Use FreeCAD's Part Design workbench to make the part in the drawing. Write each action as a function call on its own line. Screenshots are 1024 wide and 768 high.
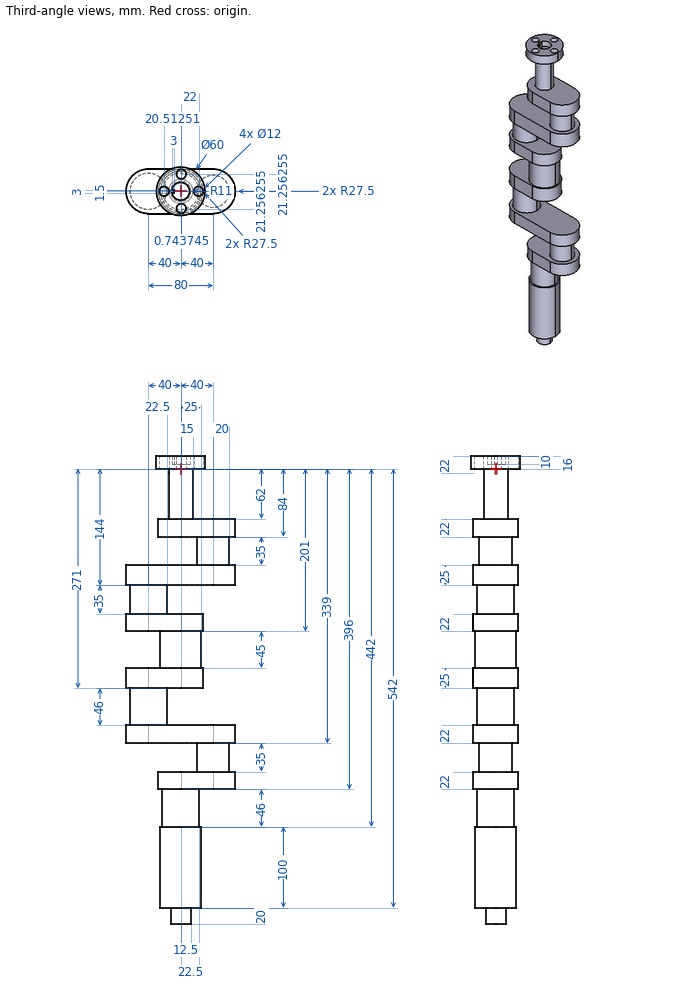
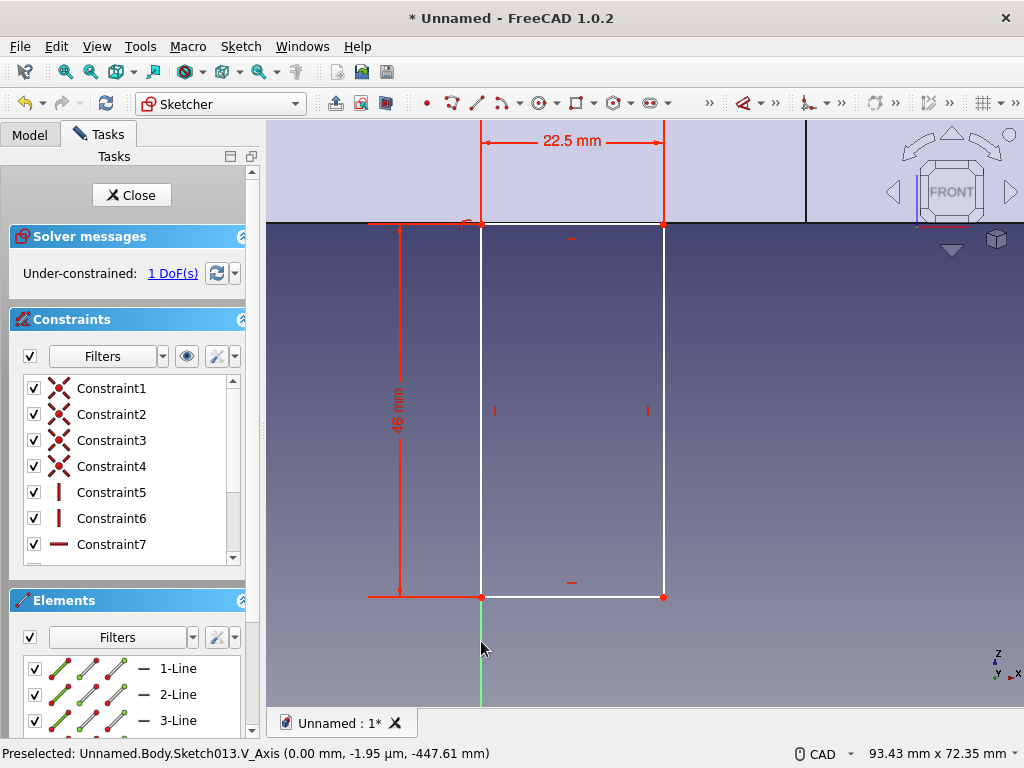
click(742, 104)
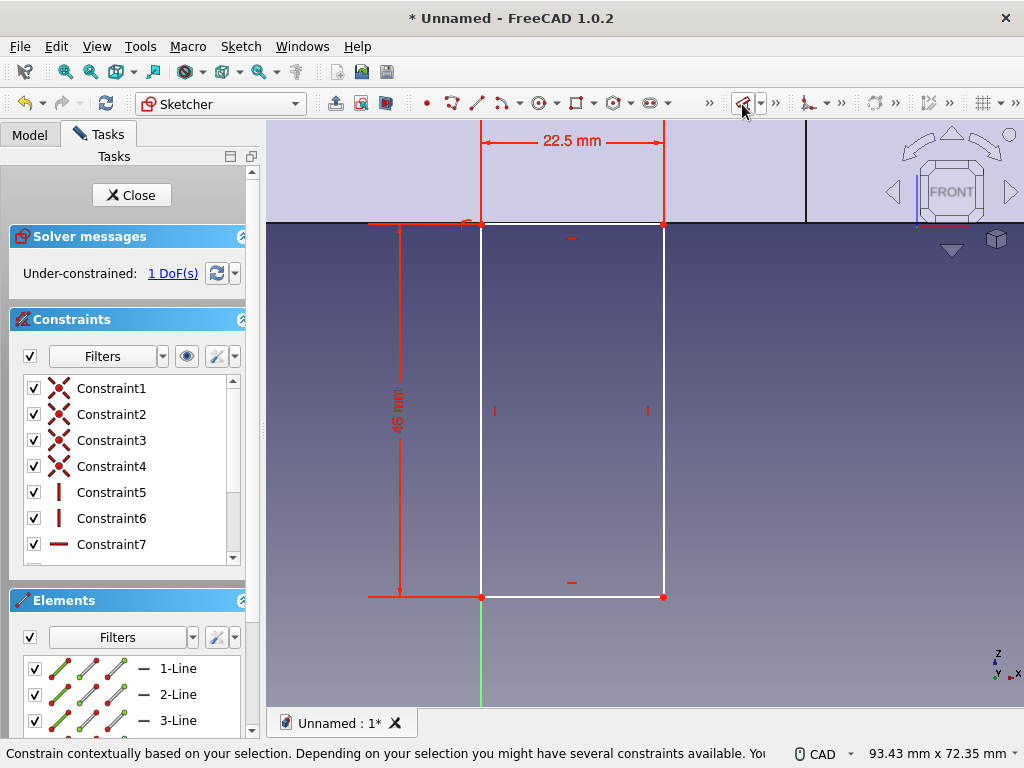
click(481, 224)
click(447, 186)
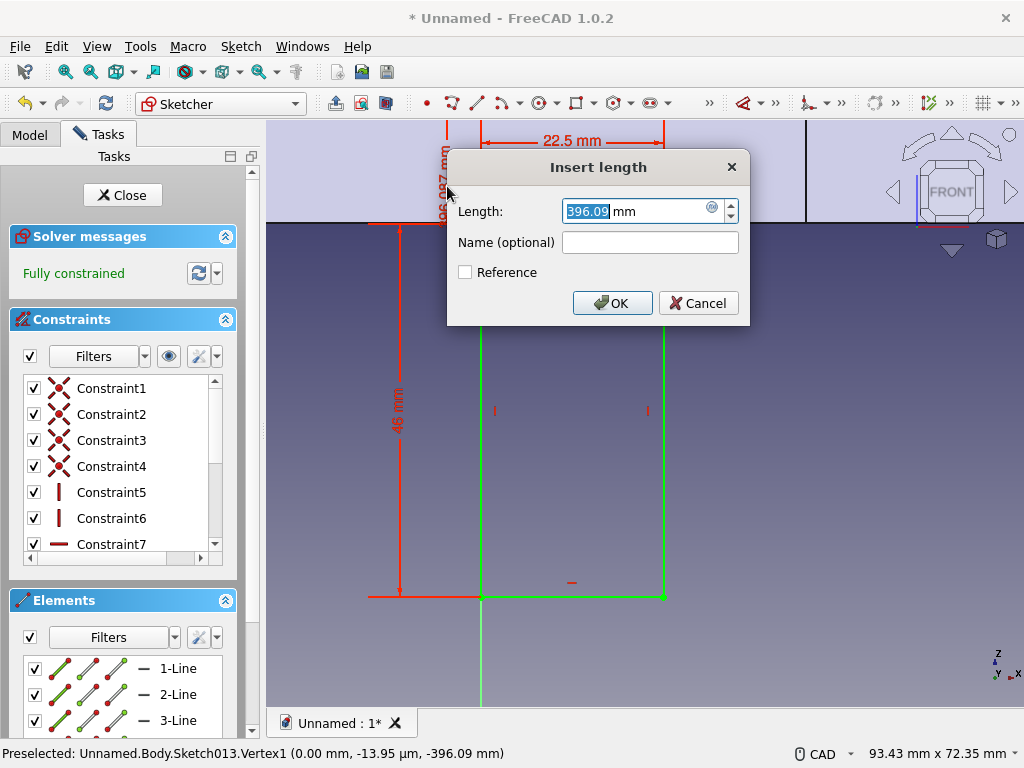
text(396)
key(Return)
key(Escape)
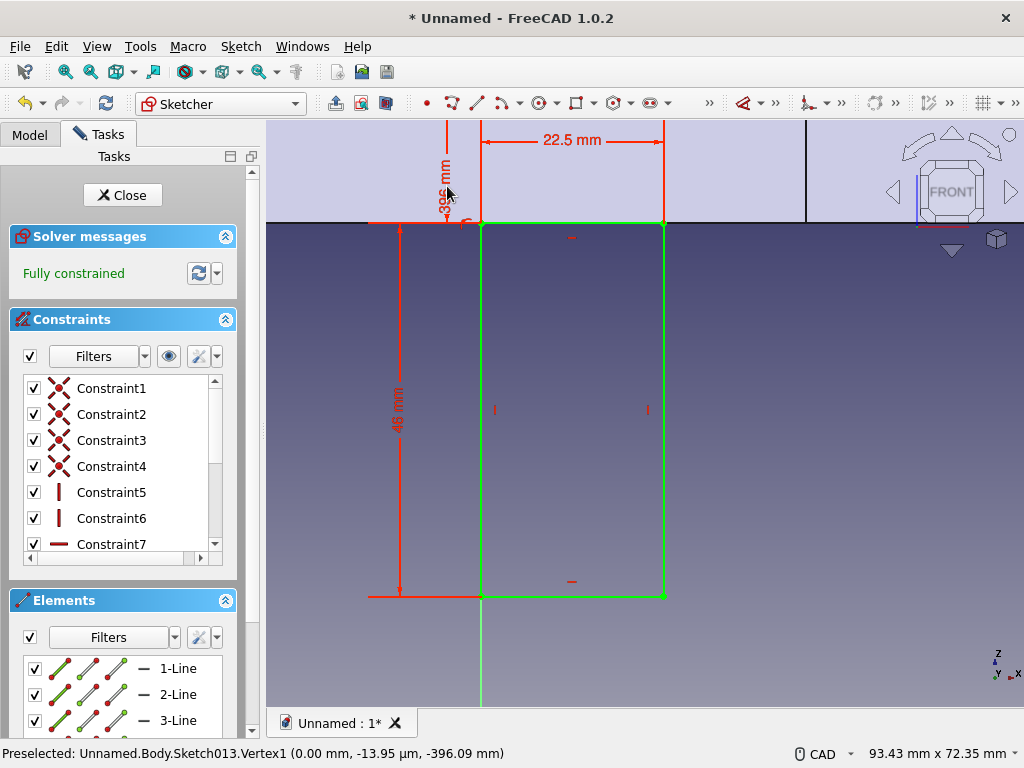
click(123, 195)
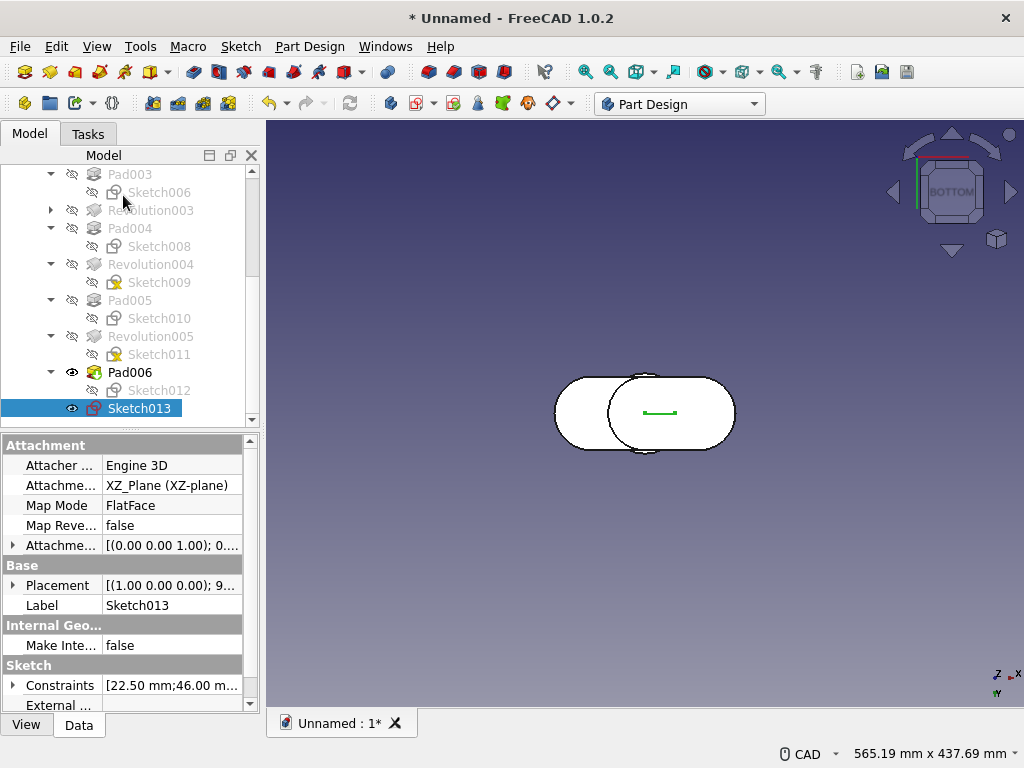
click(50, 72)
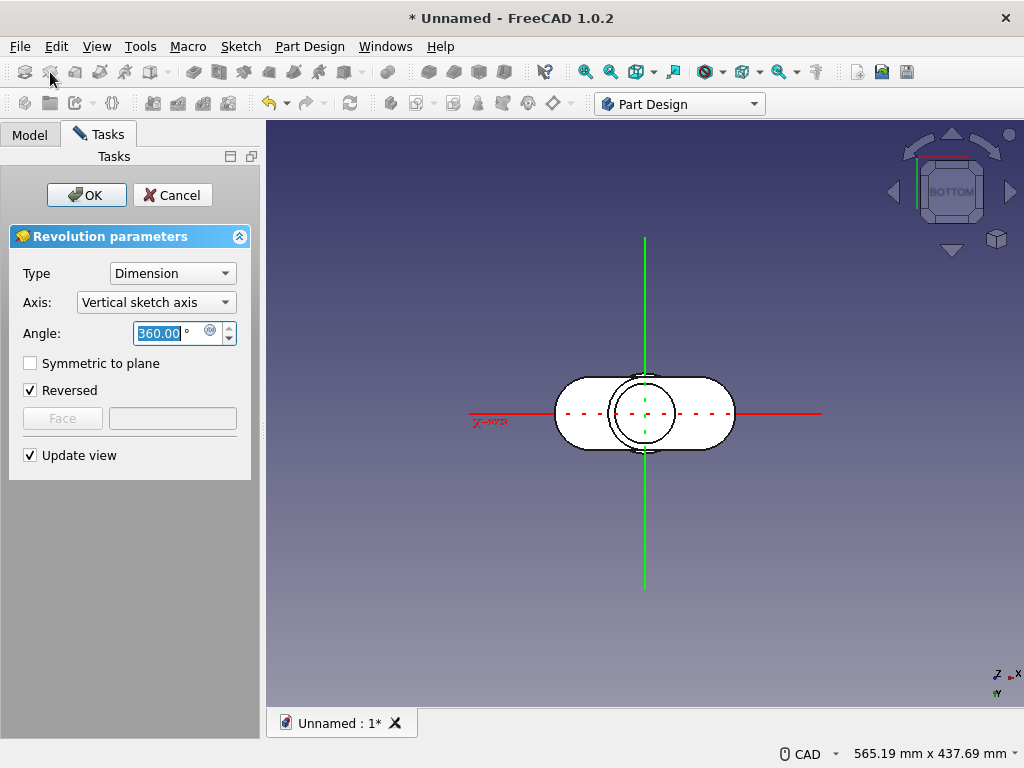
click(87, 195)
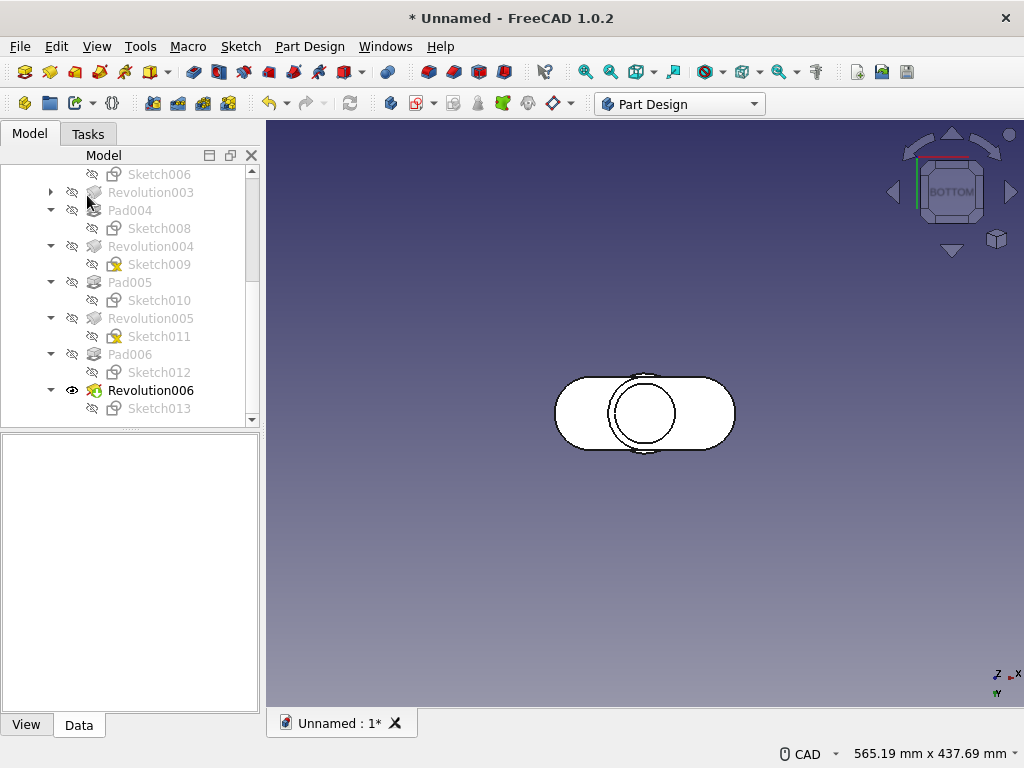
click(586, 72)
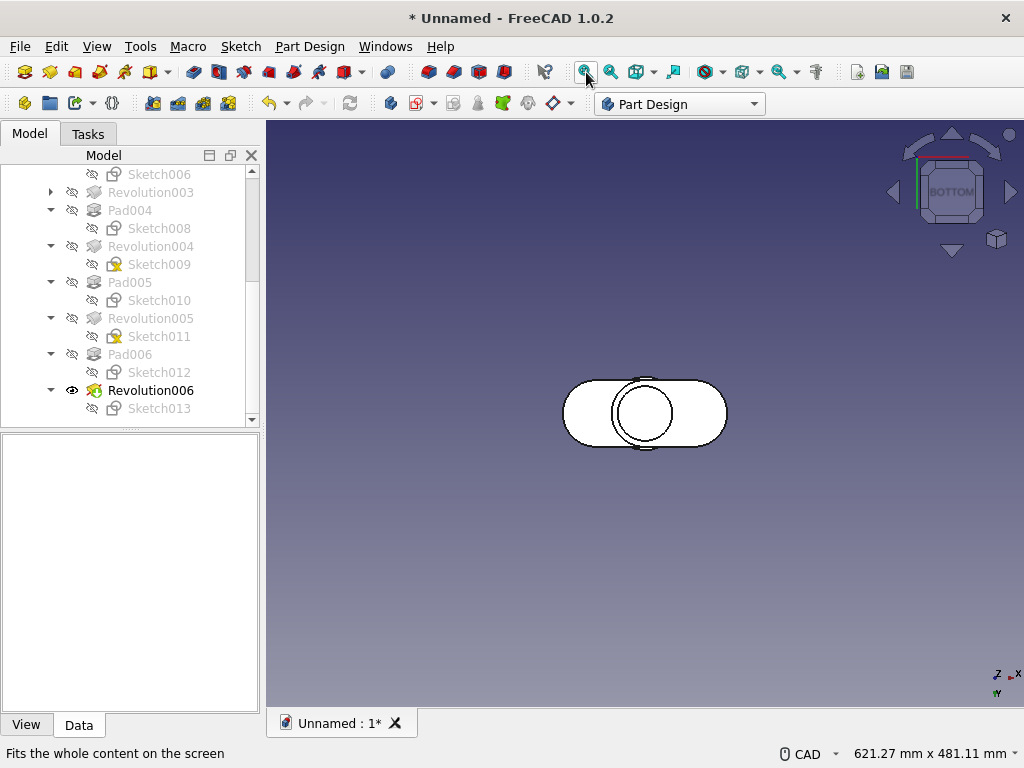
click(416, 104)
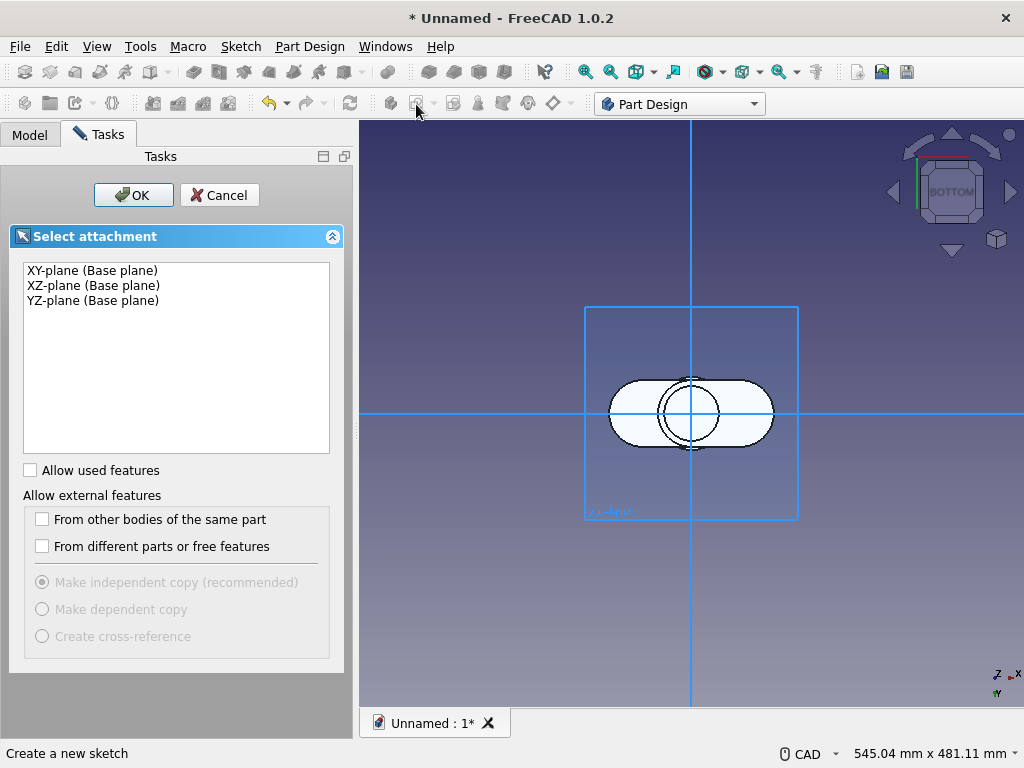
click(84, 286)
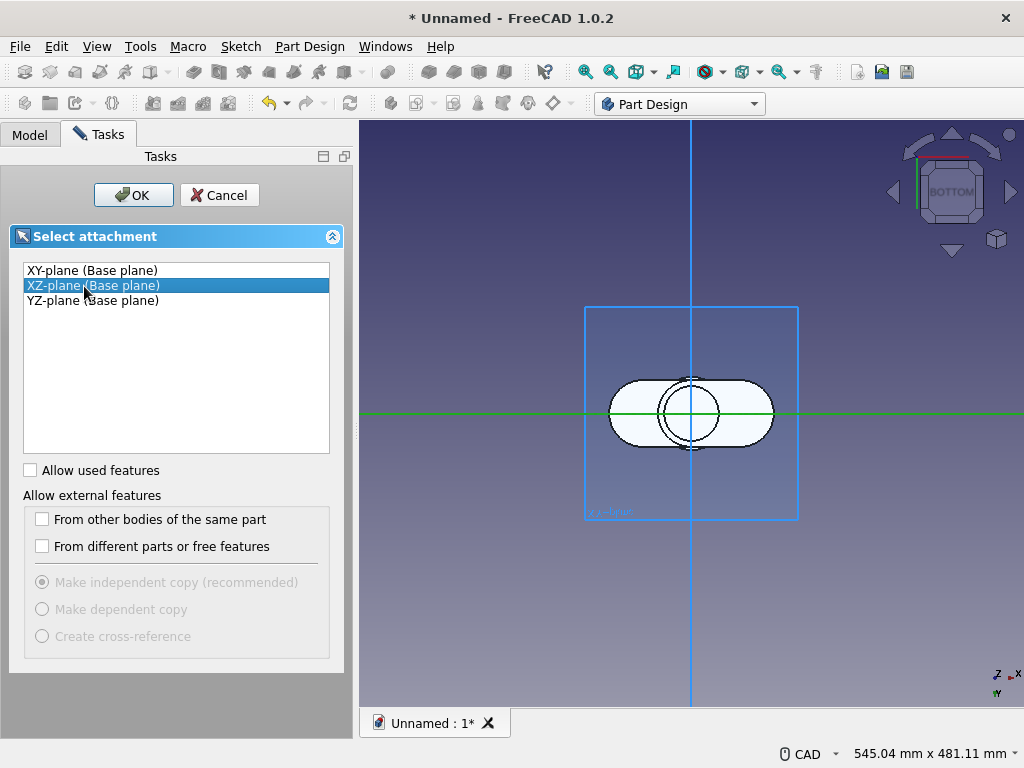
click(134, 195)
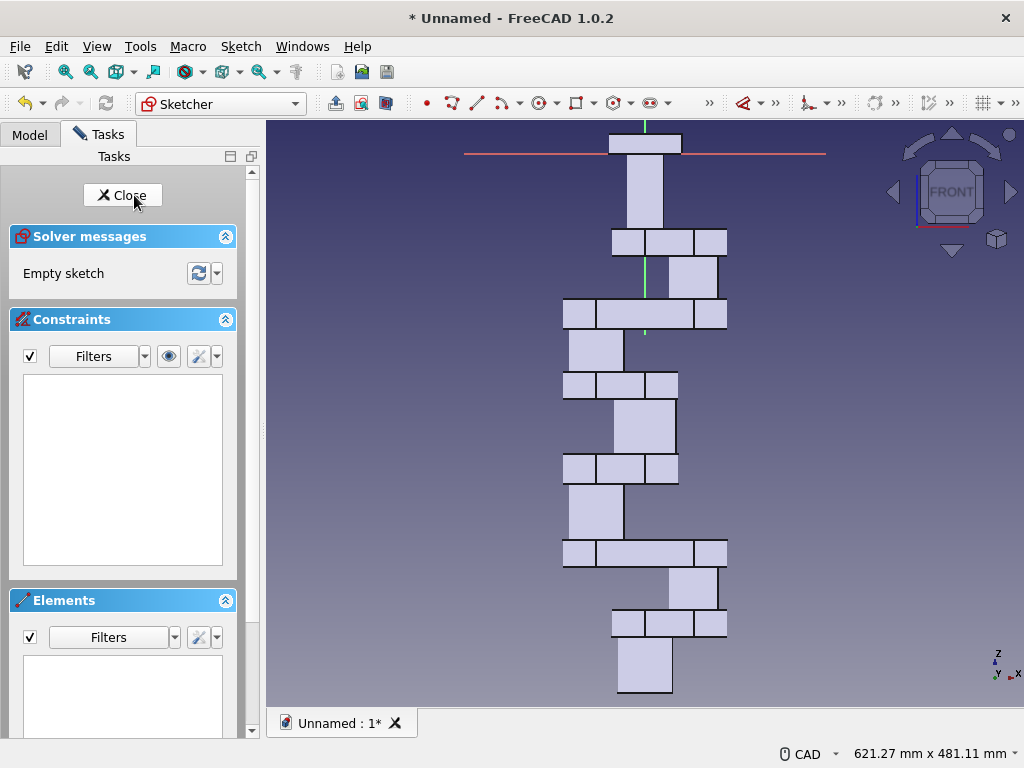
key(q)
key(s)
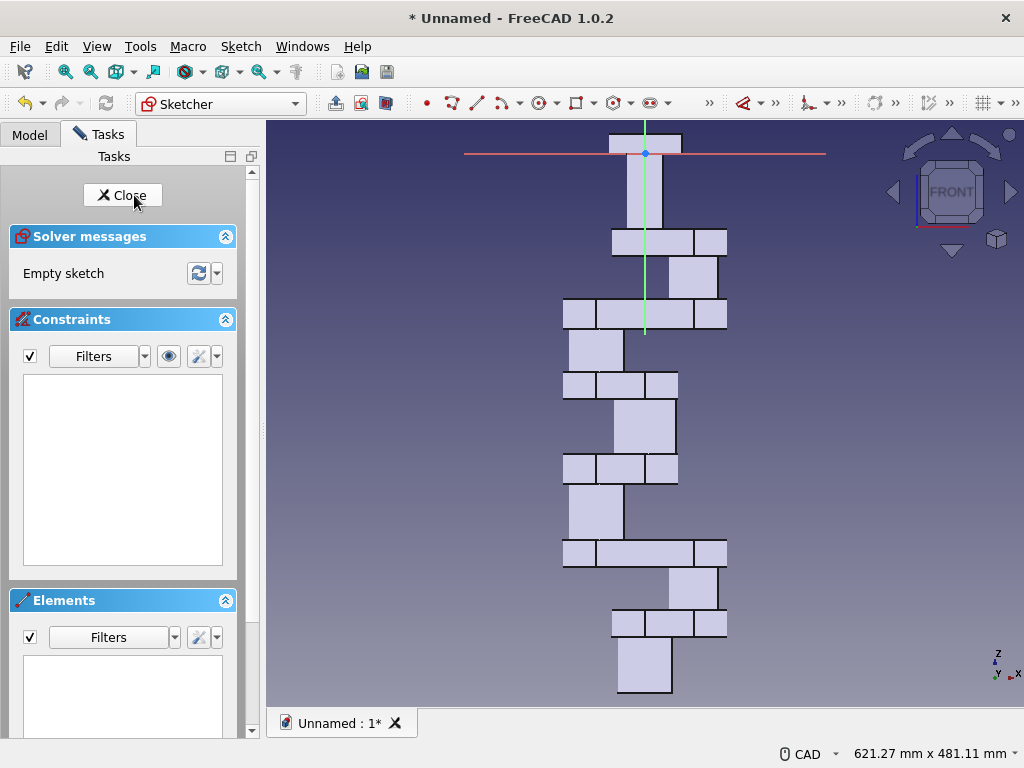
scroll(576, 414, down, 5)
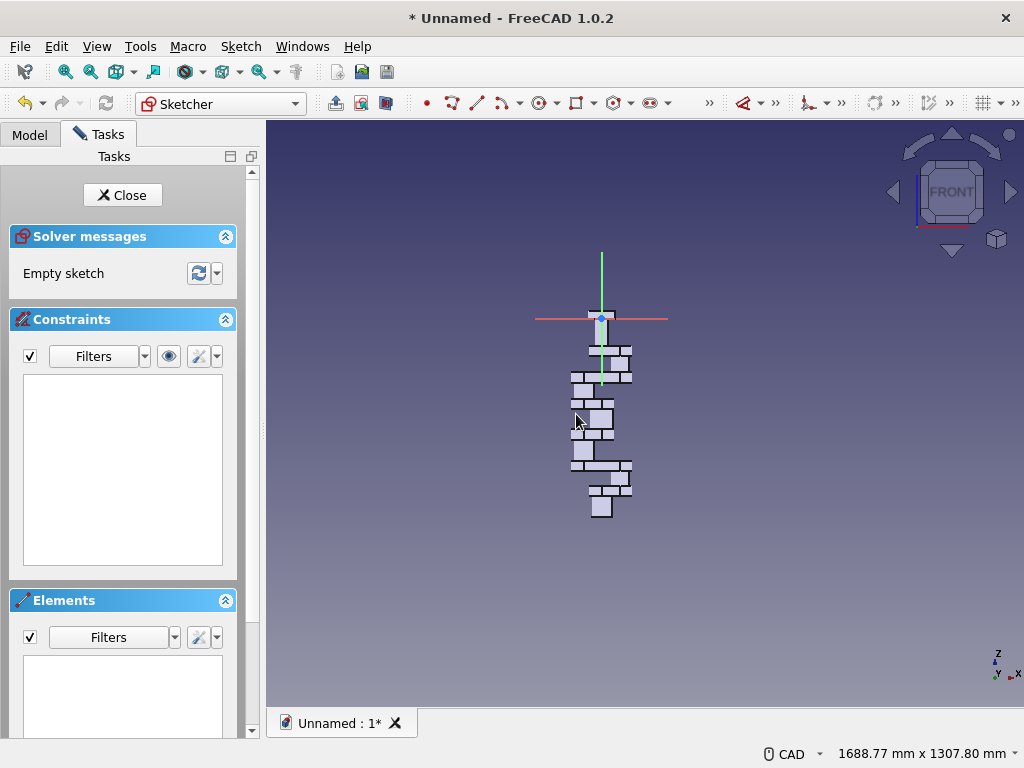
scroll(611, 555, up, 11)